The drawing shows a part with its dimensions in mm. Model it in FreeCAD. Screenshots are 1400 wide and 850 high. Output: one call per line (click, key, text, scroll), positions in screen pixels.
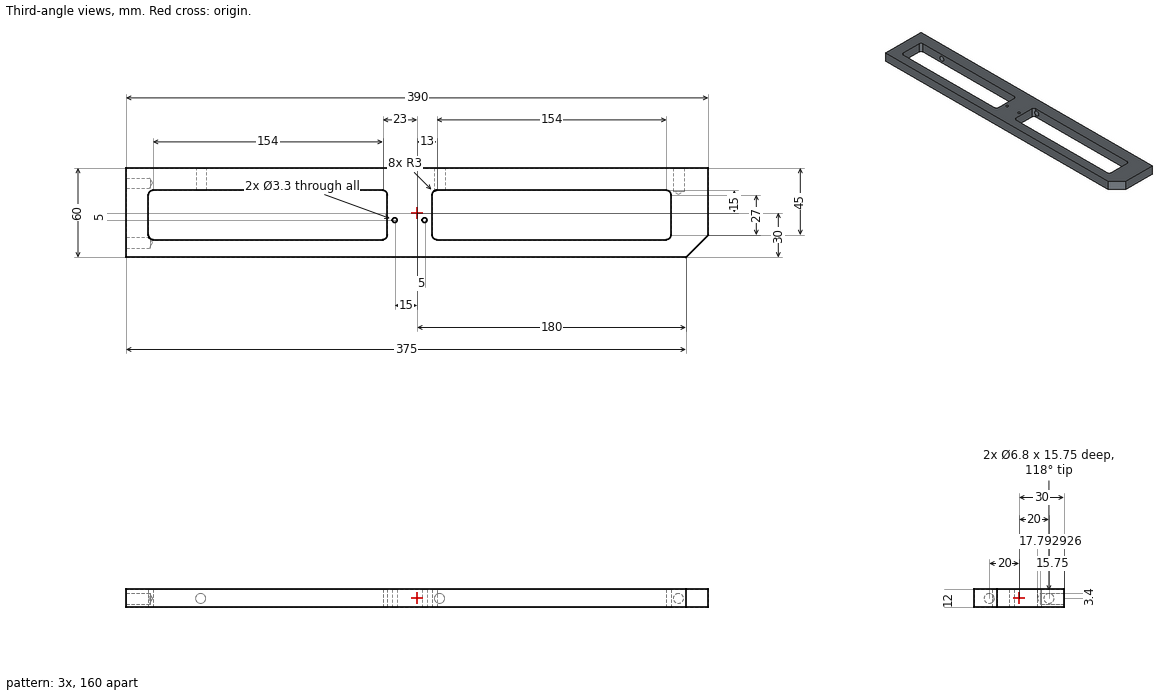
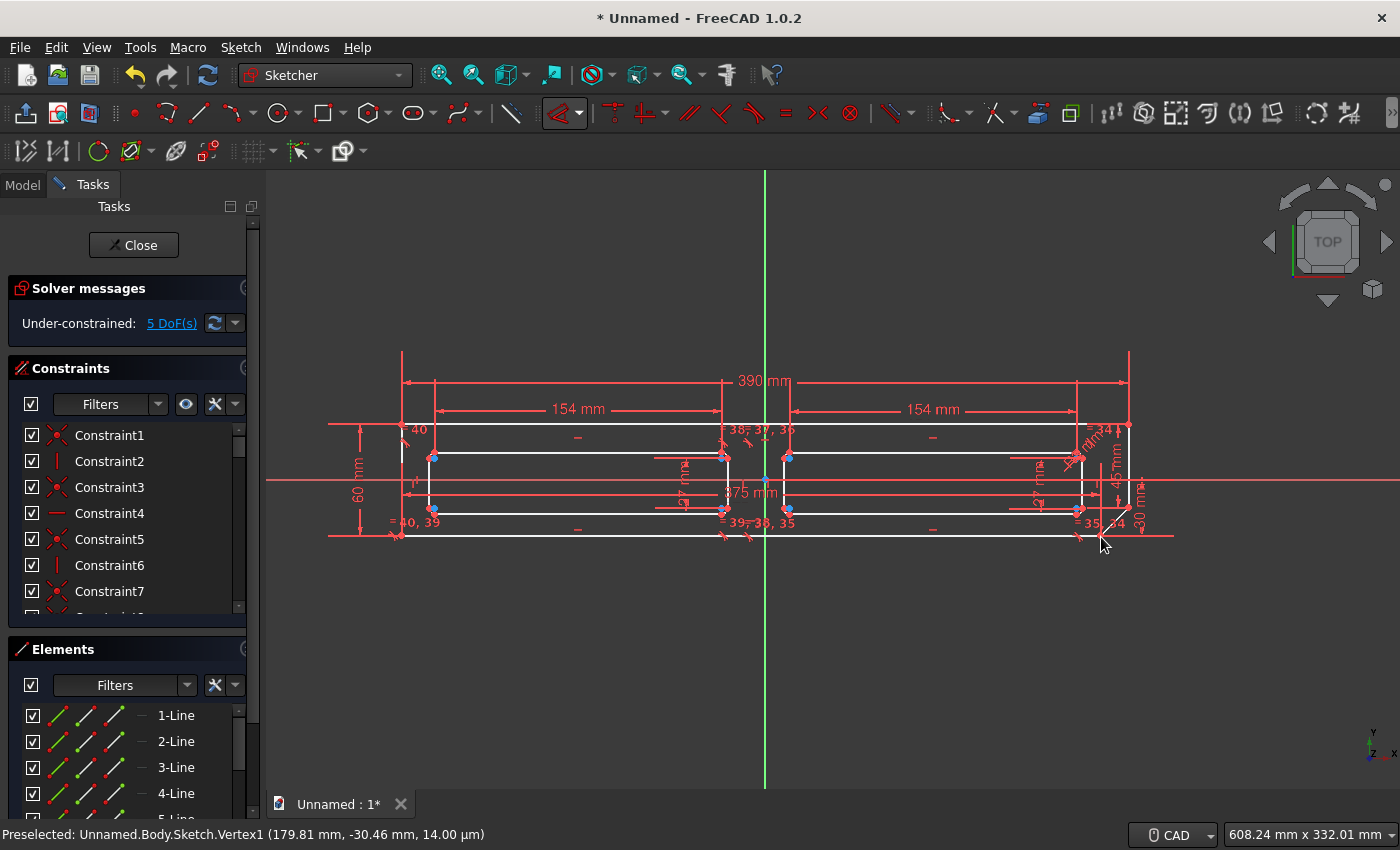
scroll(790, 453, up, 4)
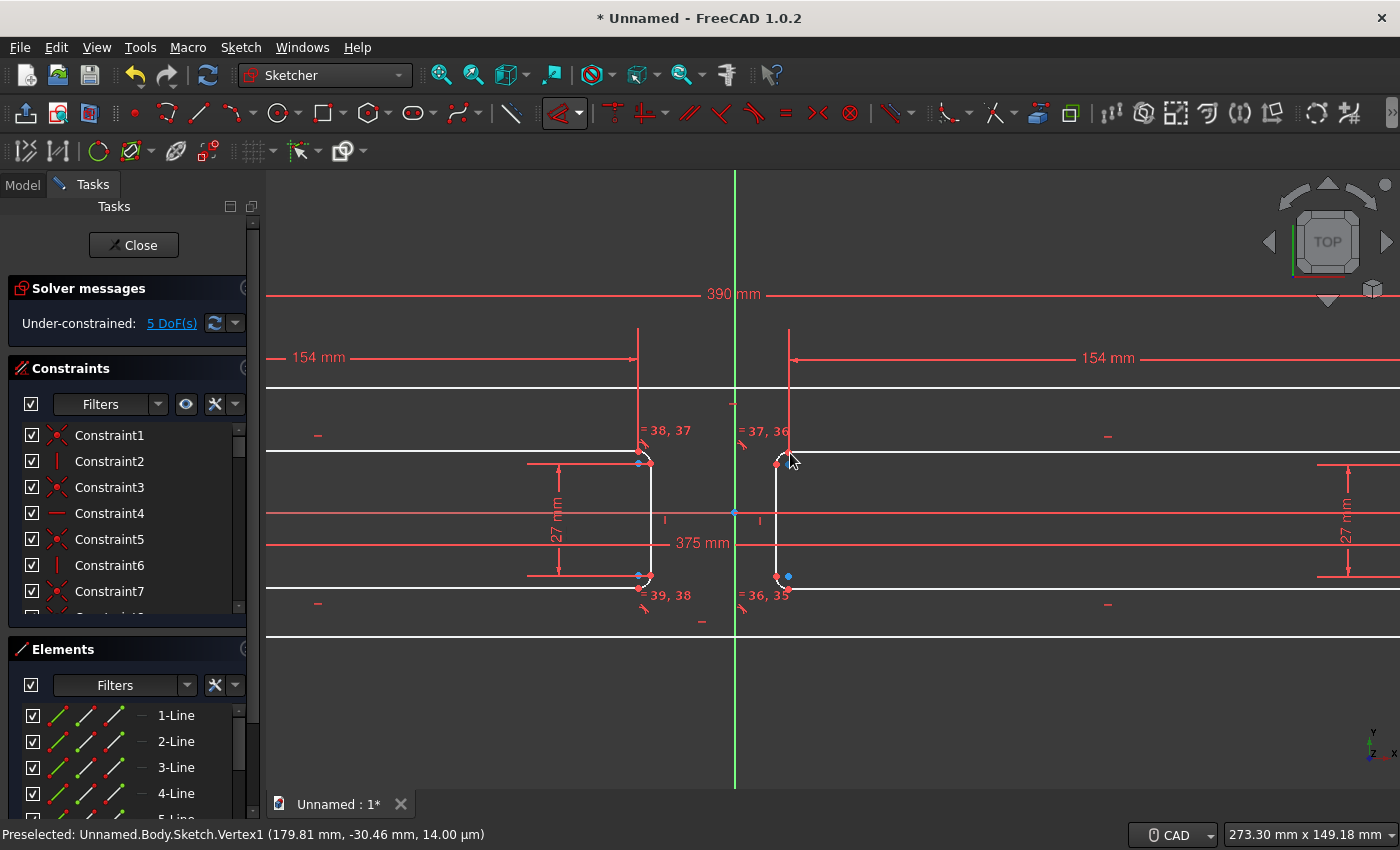
click(789, 452)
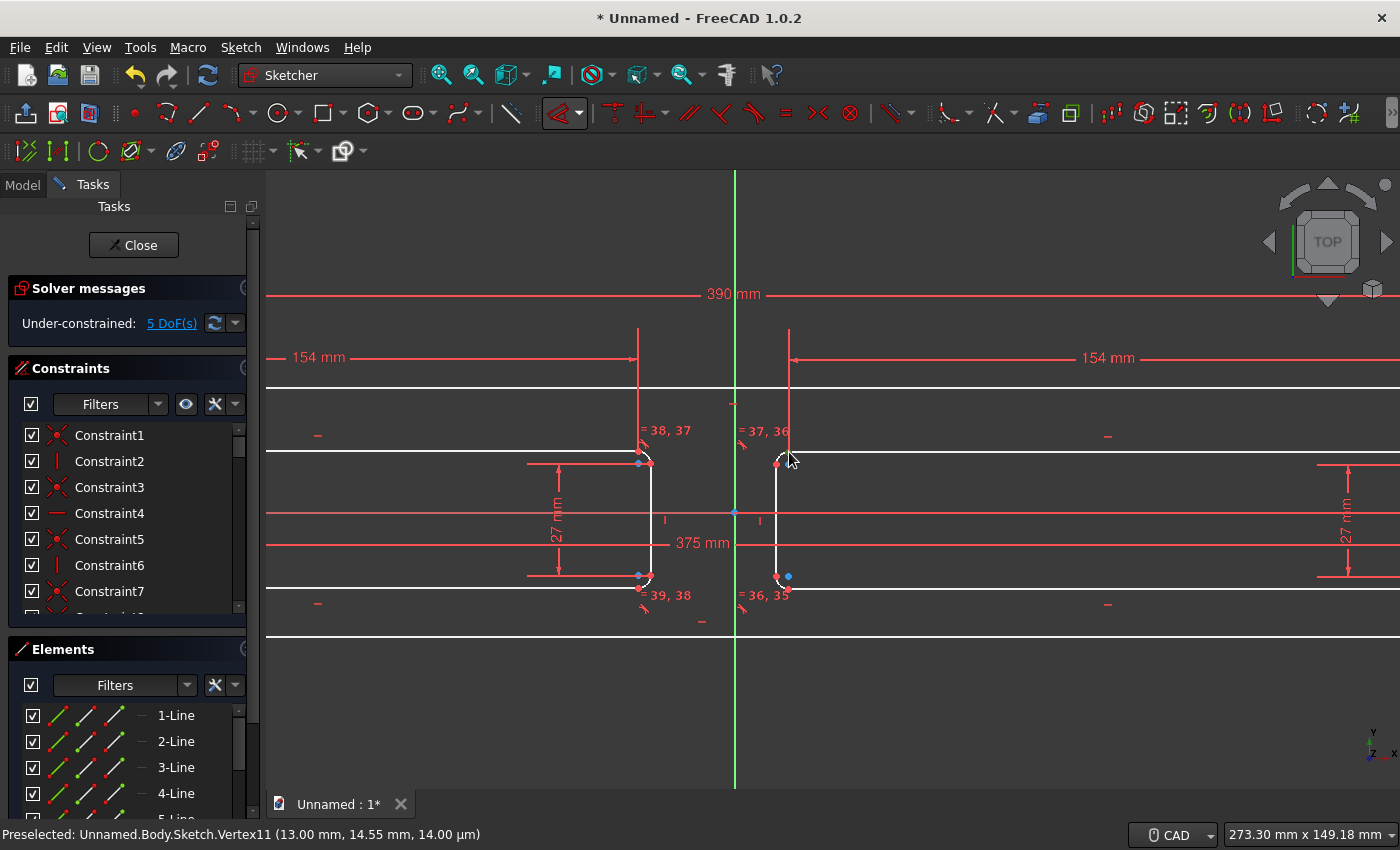
click(582, 114)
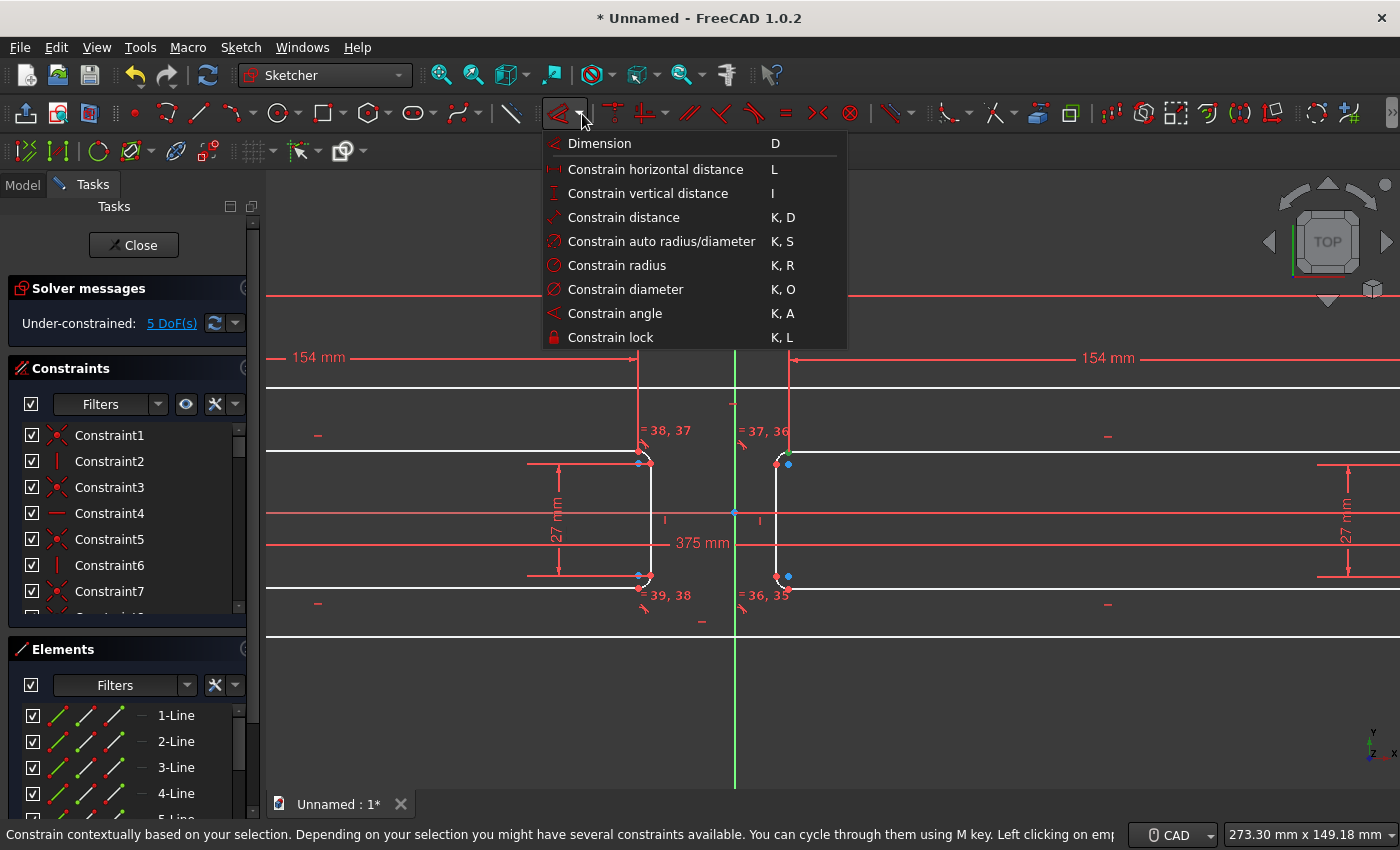
click(695, 169)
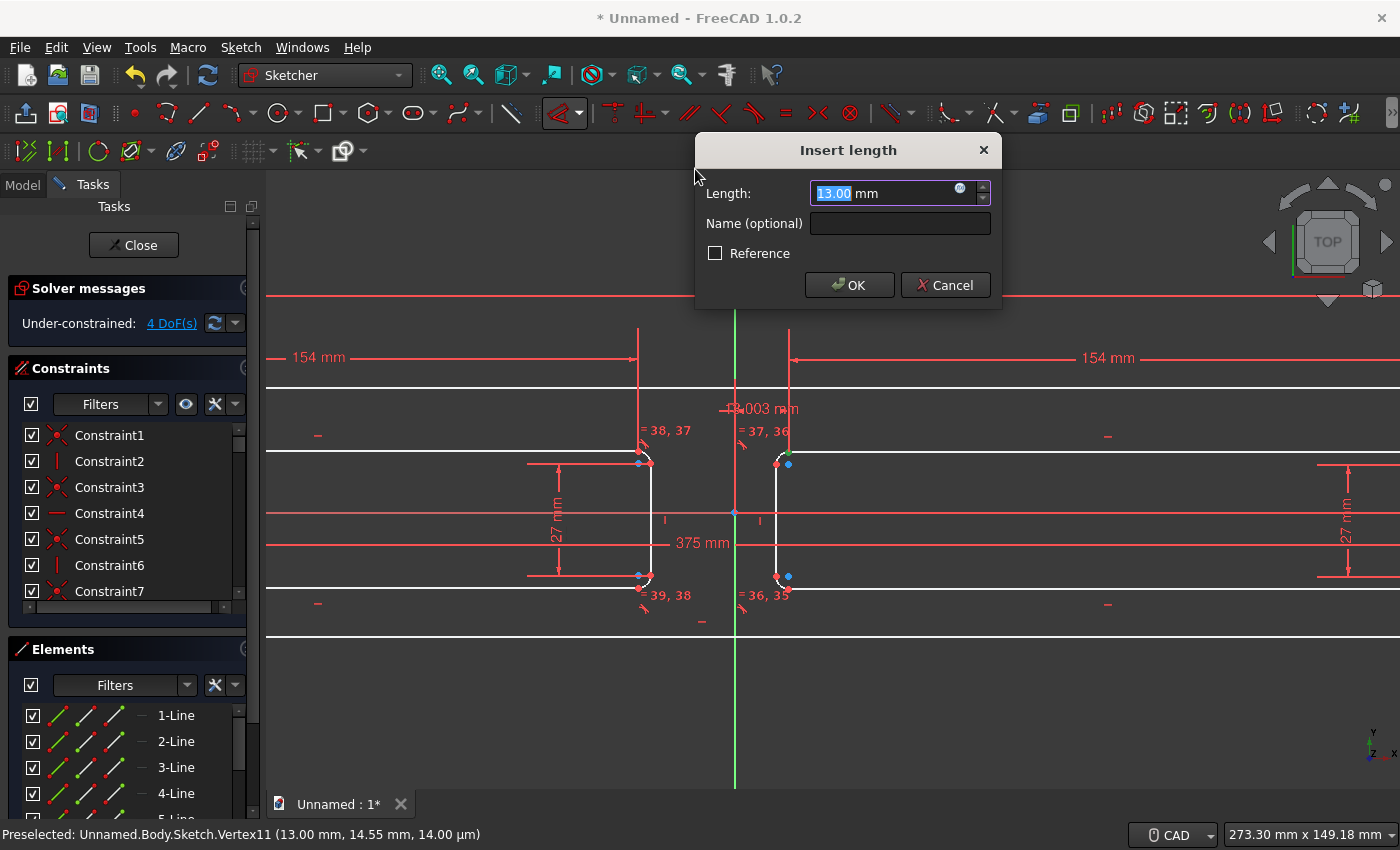
text(13)
key(Return)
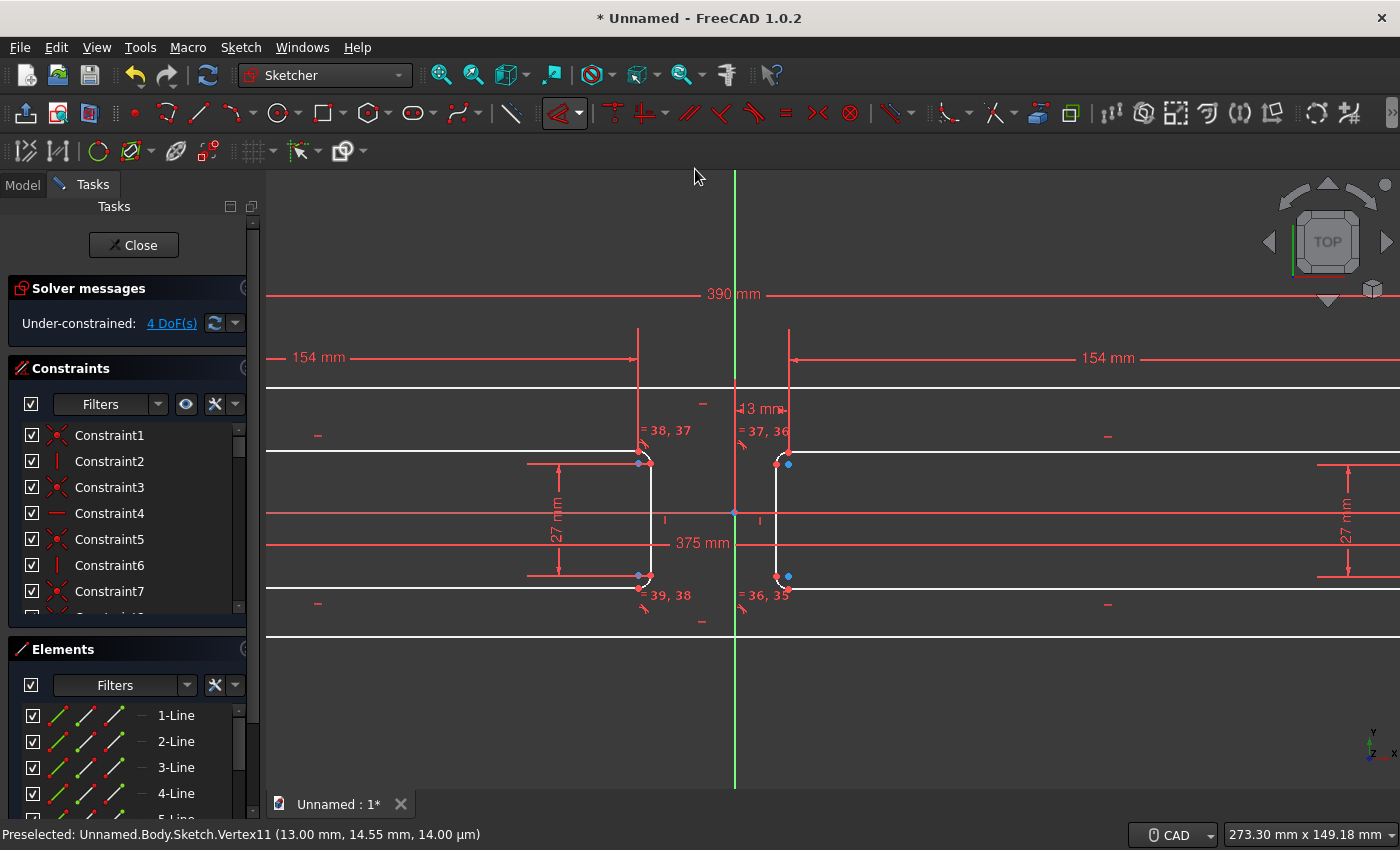
click(789, 452)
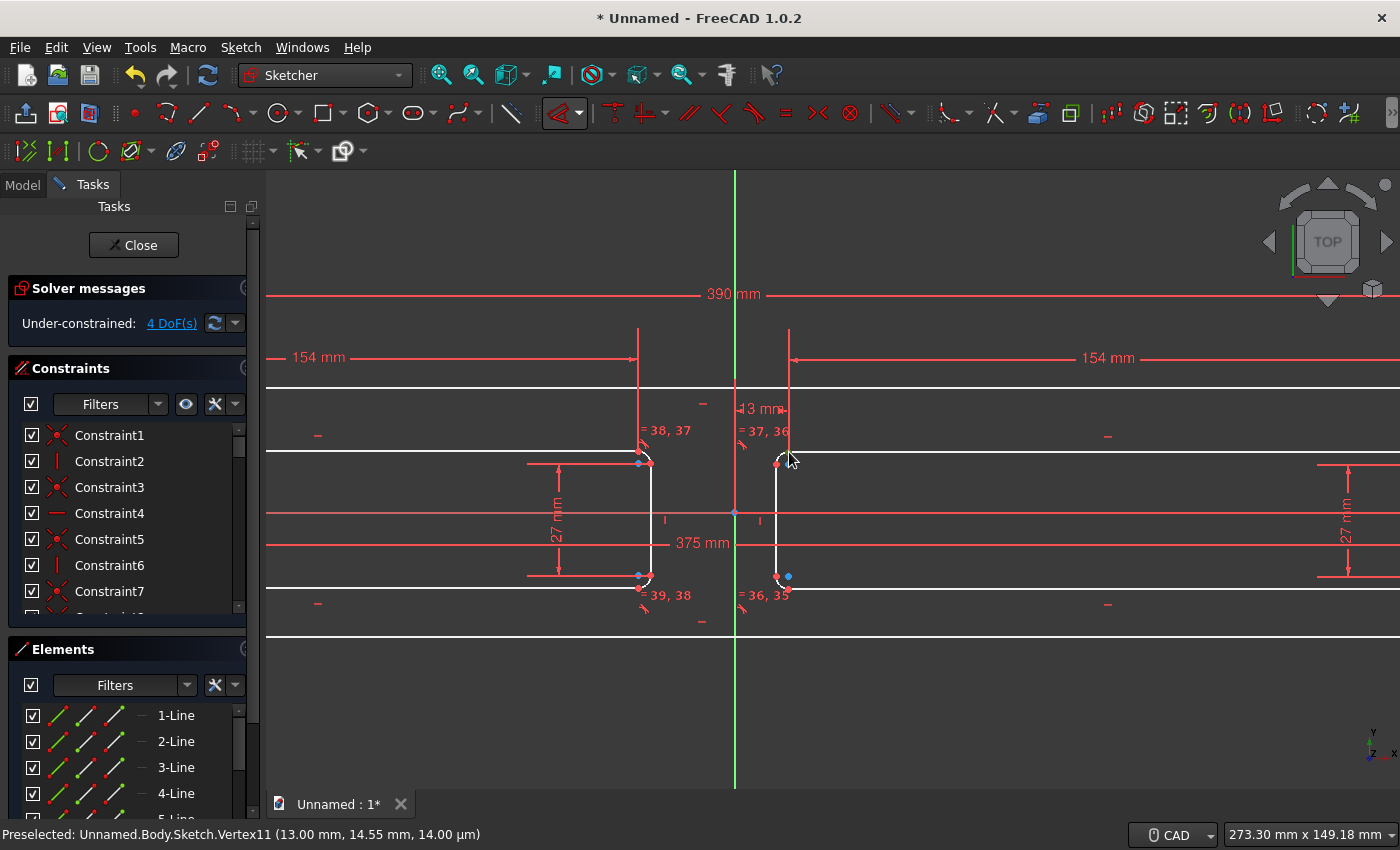
click(582, 114)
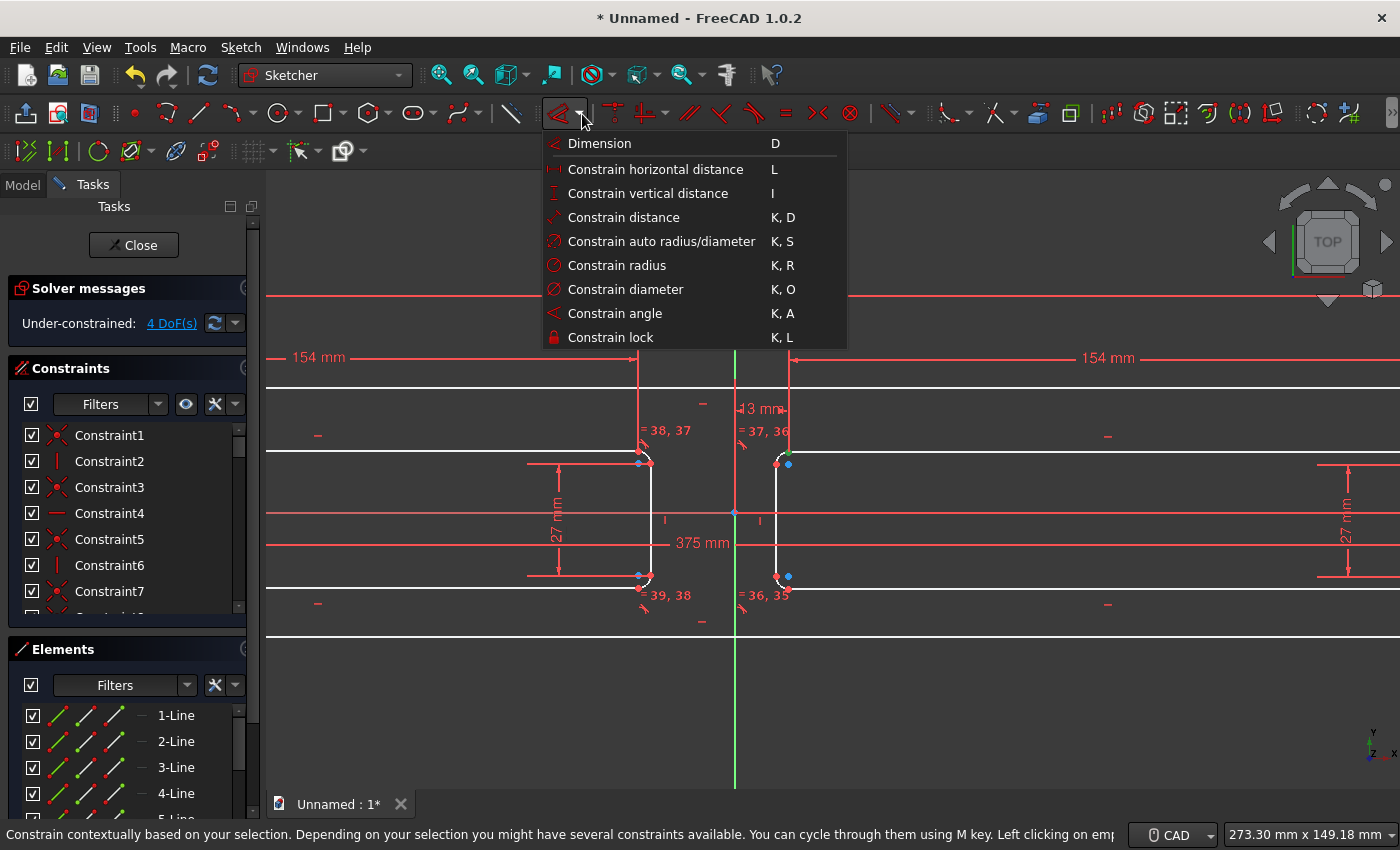
click(695, 193)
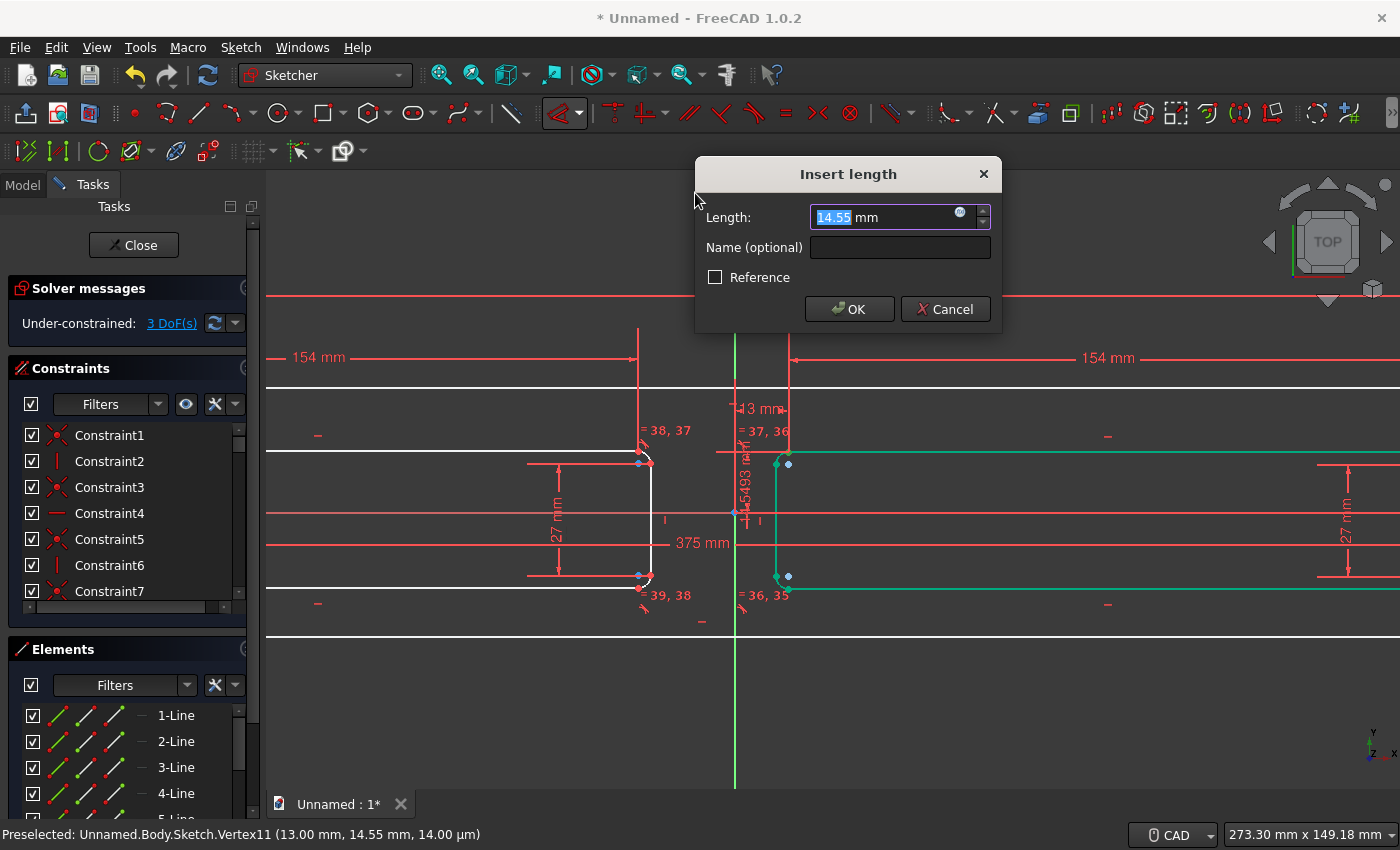
text(15)
key(Return)